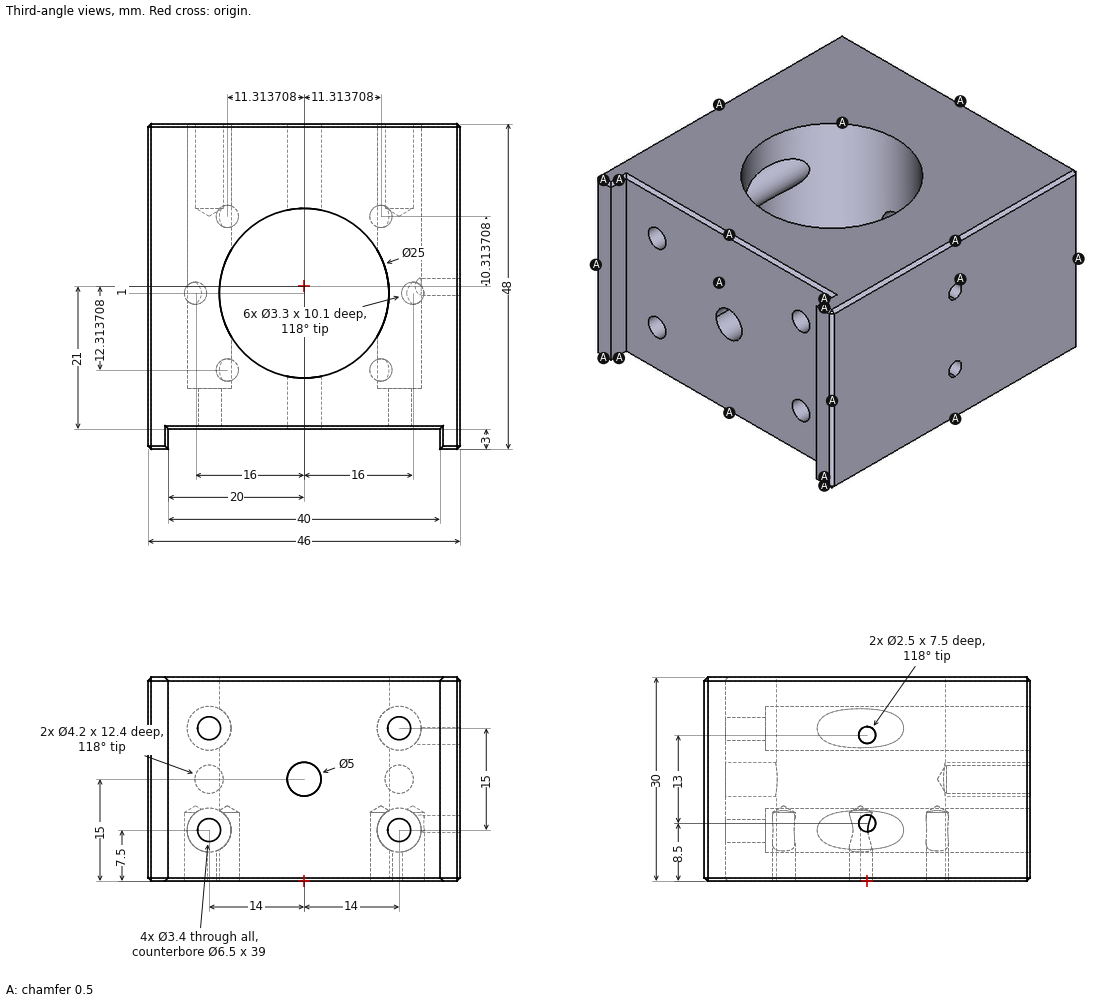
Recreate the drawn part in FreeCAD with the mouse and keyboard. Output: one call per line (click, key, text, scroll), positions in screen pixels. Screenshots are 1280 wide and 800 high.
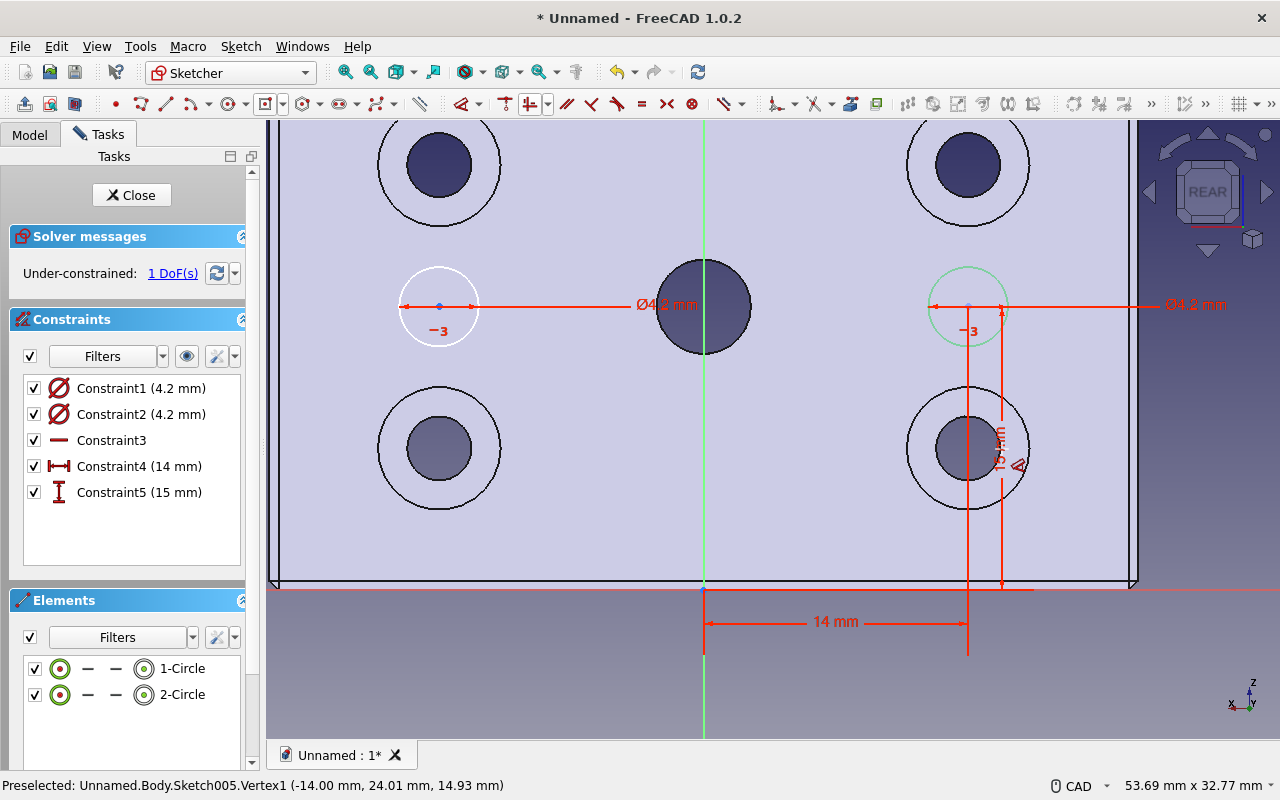
click(439, 307)
click(571, 624)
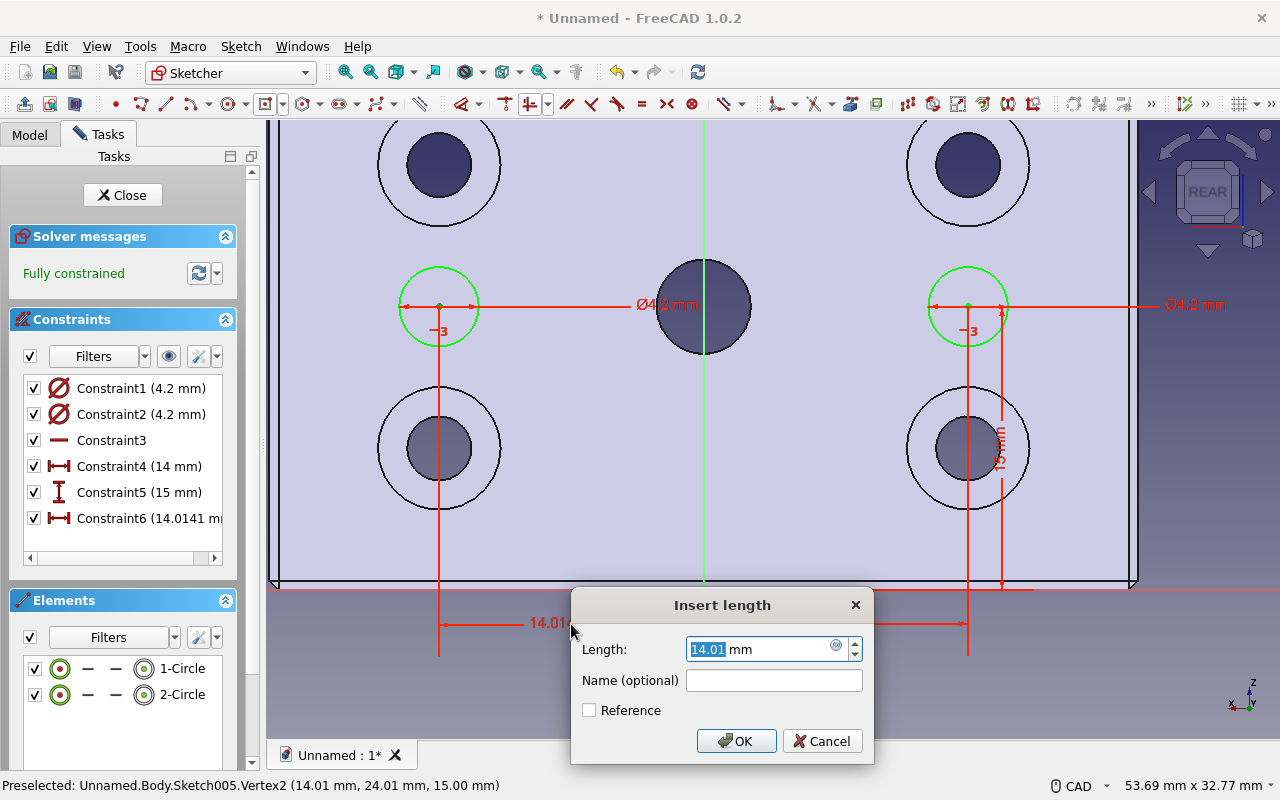
text(14)
key(Return)
key(Escape)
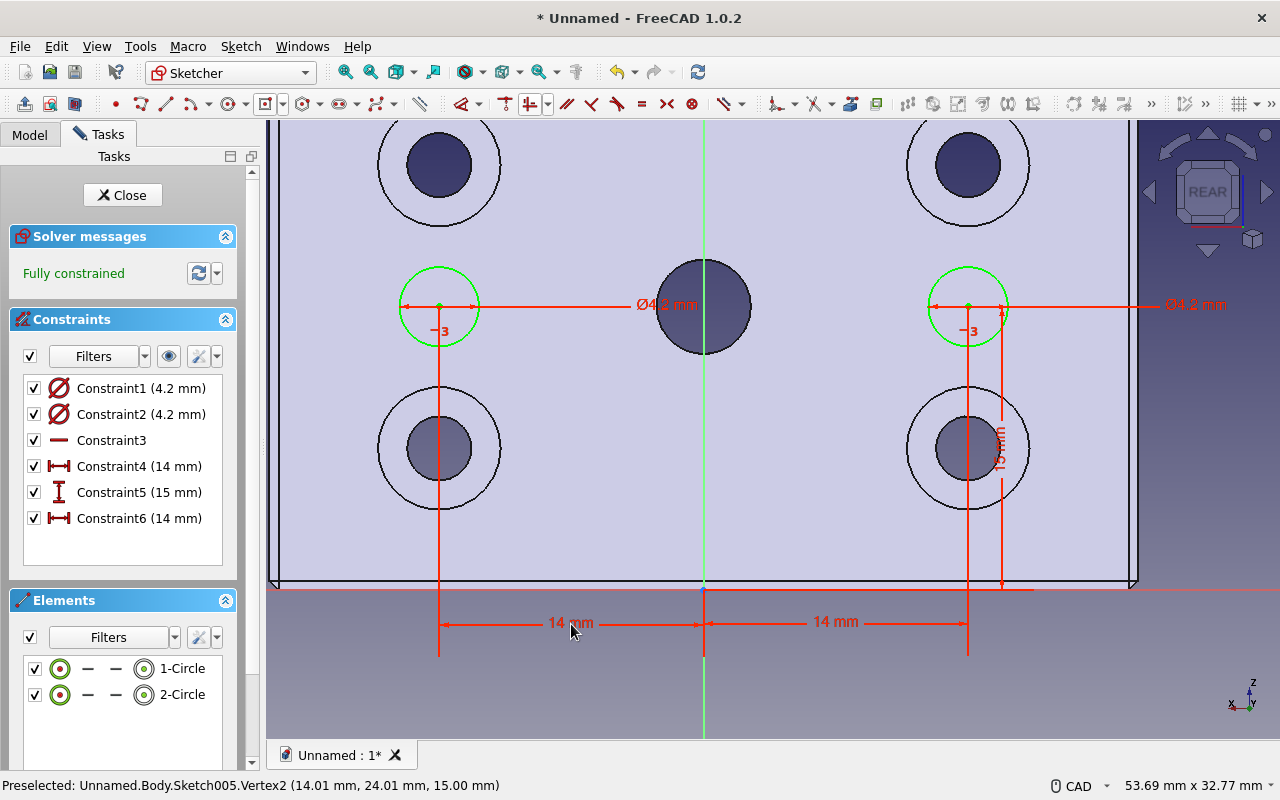
click(123, 195)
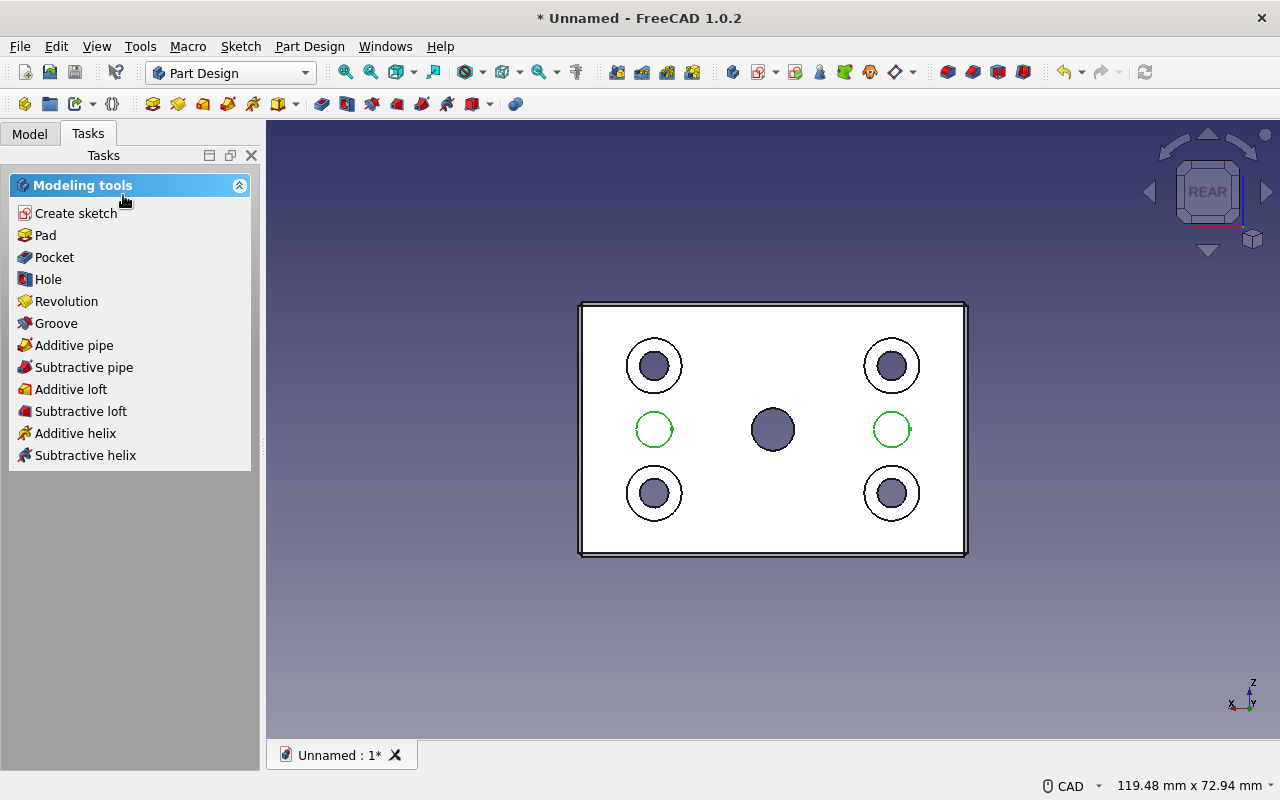
click(347, 104)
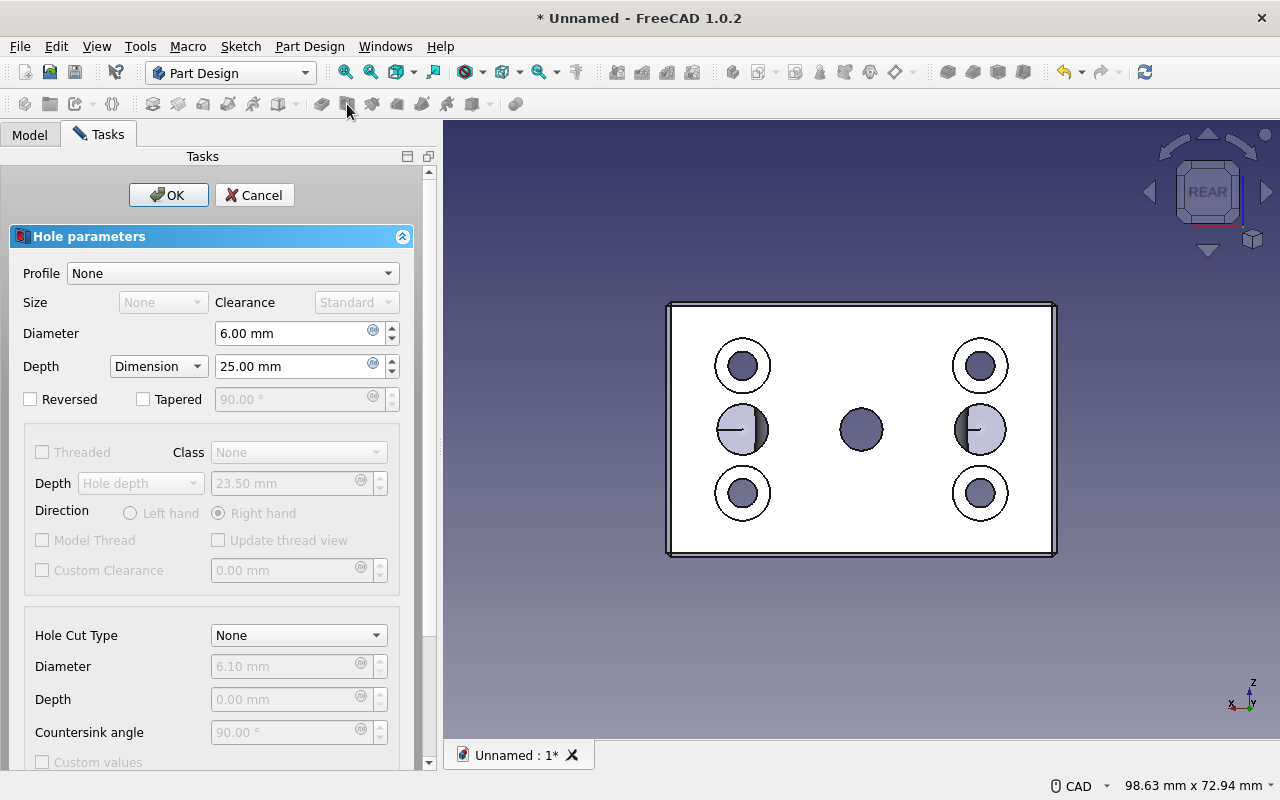
triple_click(300, 334)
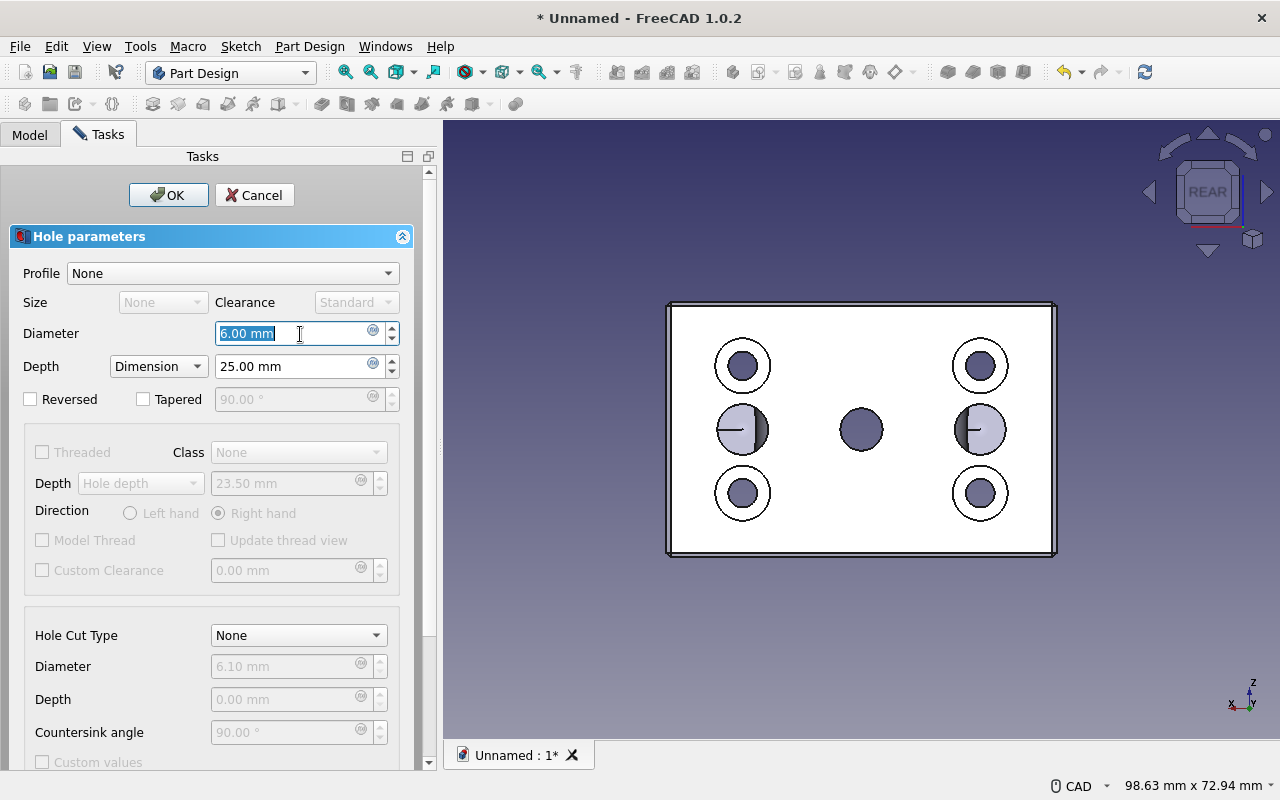
text(4.2)
key(Tab)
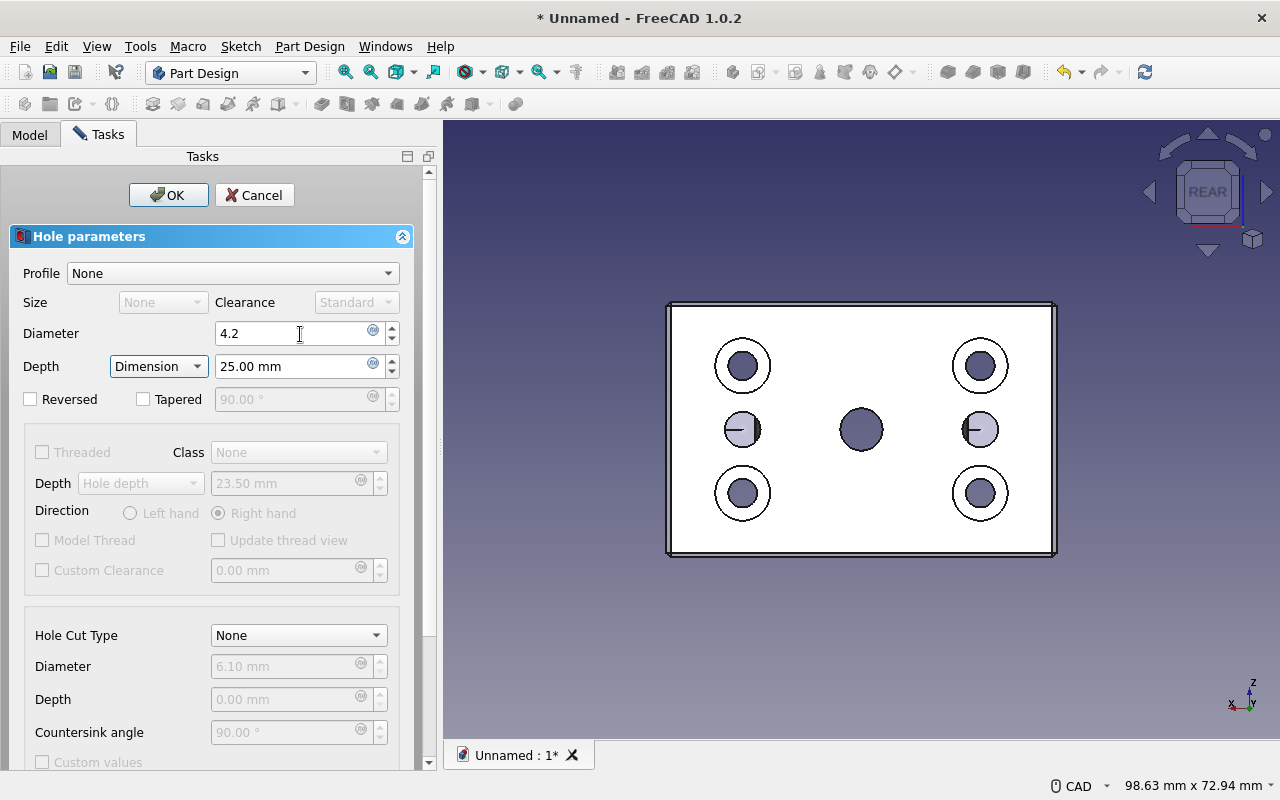
triple_click(300, 366)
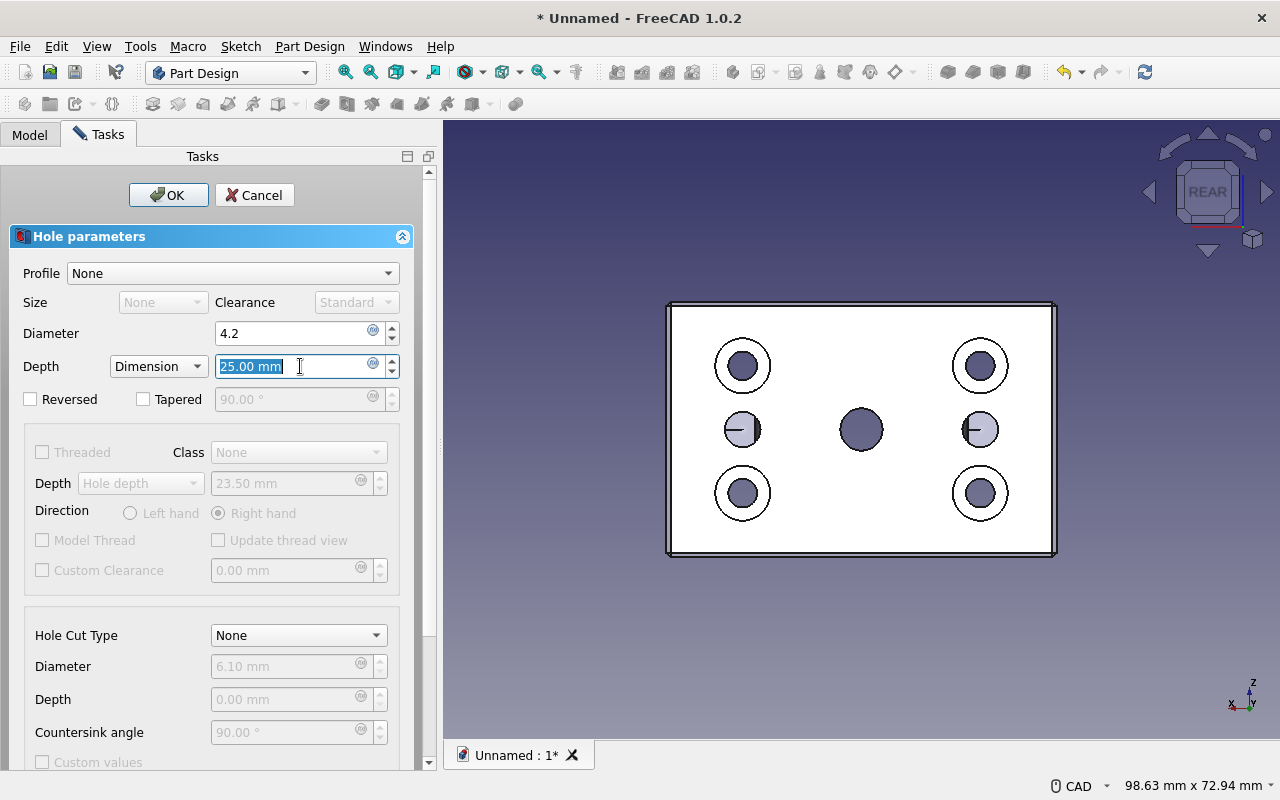
text(12.4)
key(Tab)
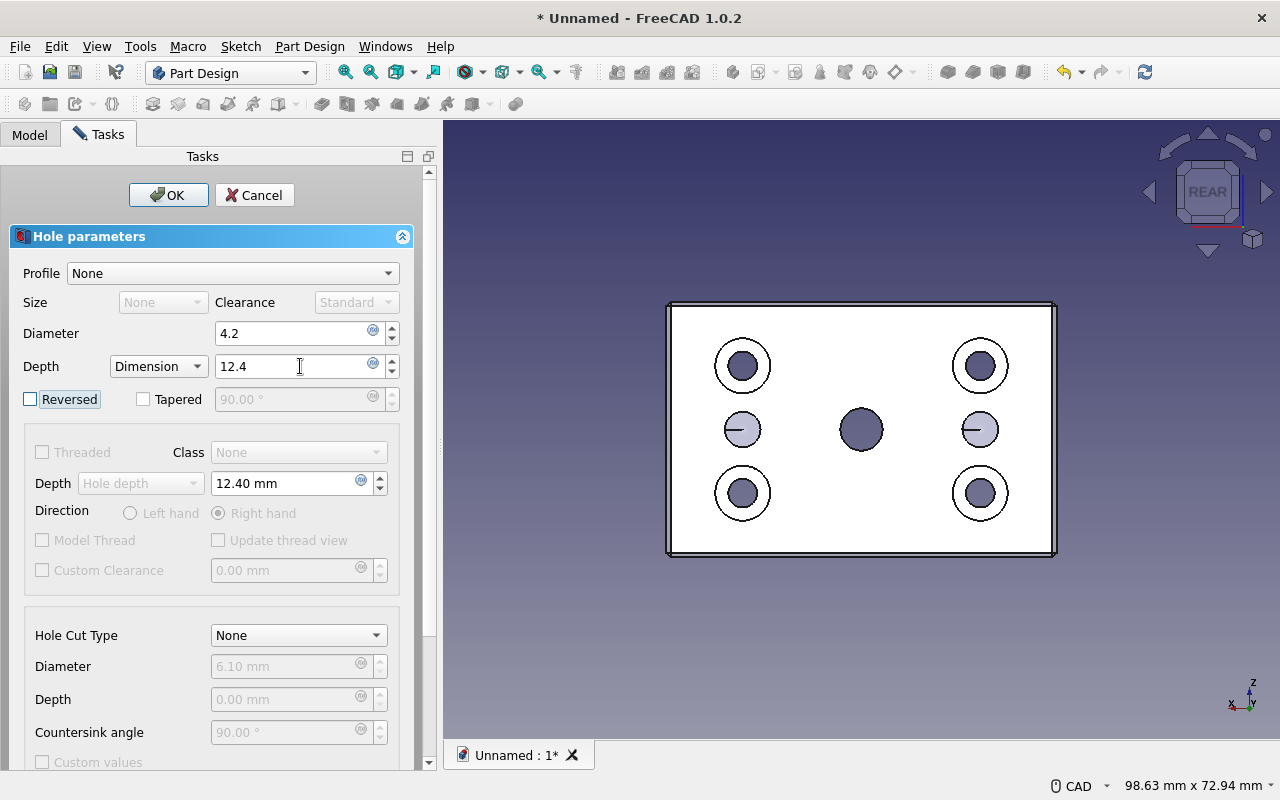
click(169, 195)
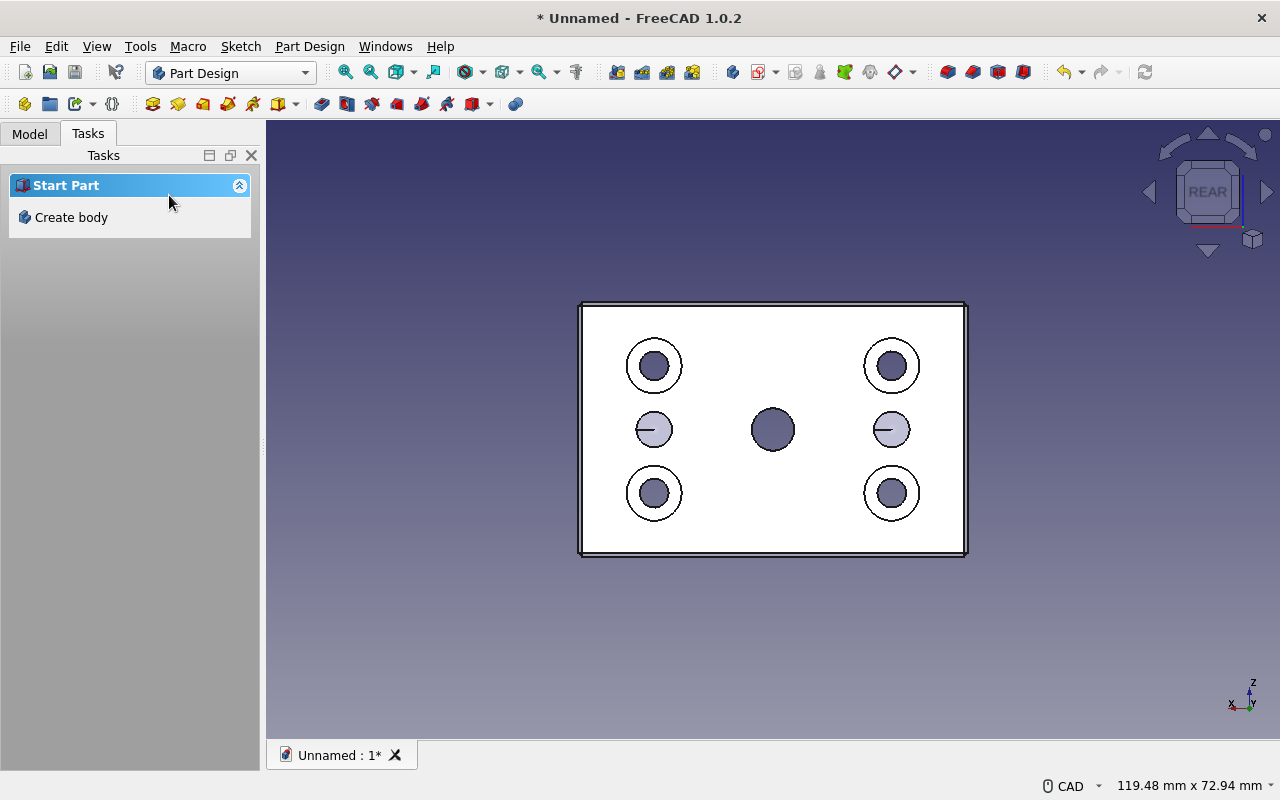
click(346, 72)